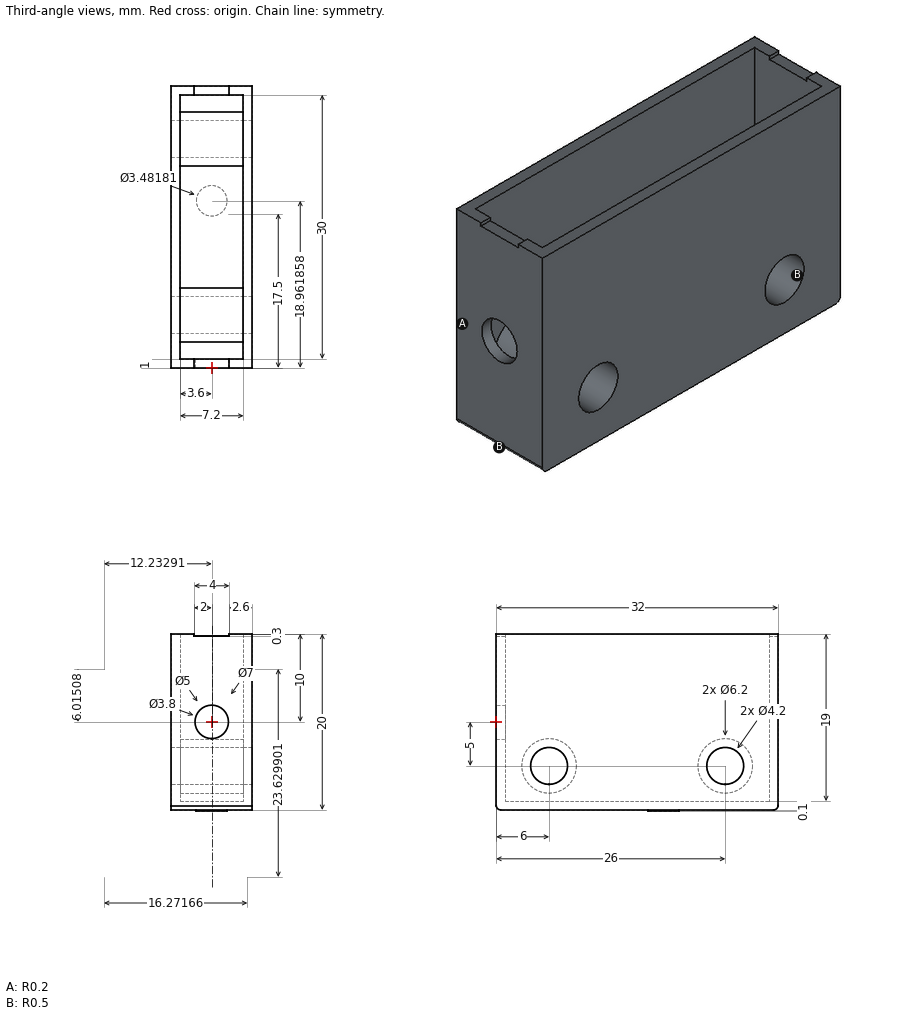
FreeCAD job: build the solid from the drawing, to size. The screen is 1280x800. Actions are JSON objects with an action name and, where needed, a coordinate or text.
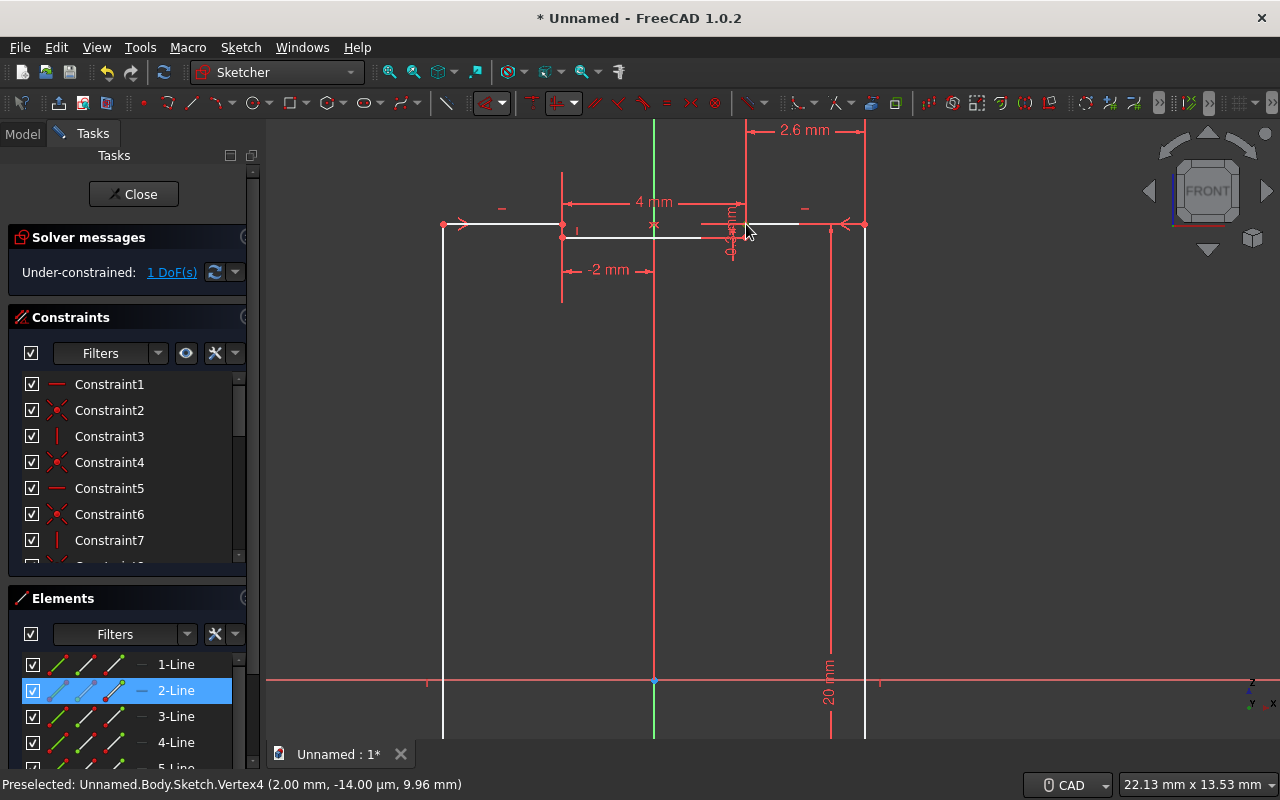
{"action": "left_click", "coordinate": [504, 104]}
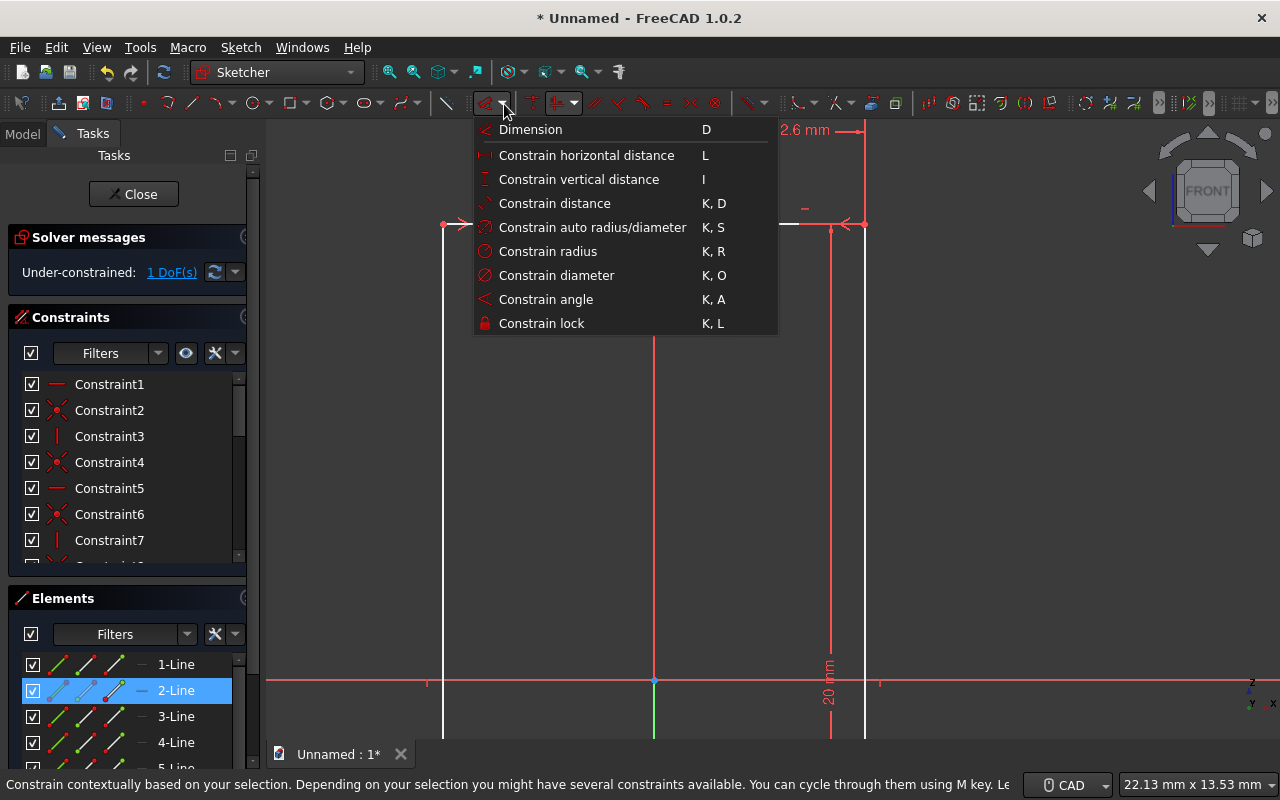
{"action": "left_click", "coordinate": [626, 179]}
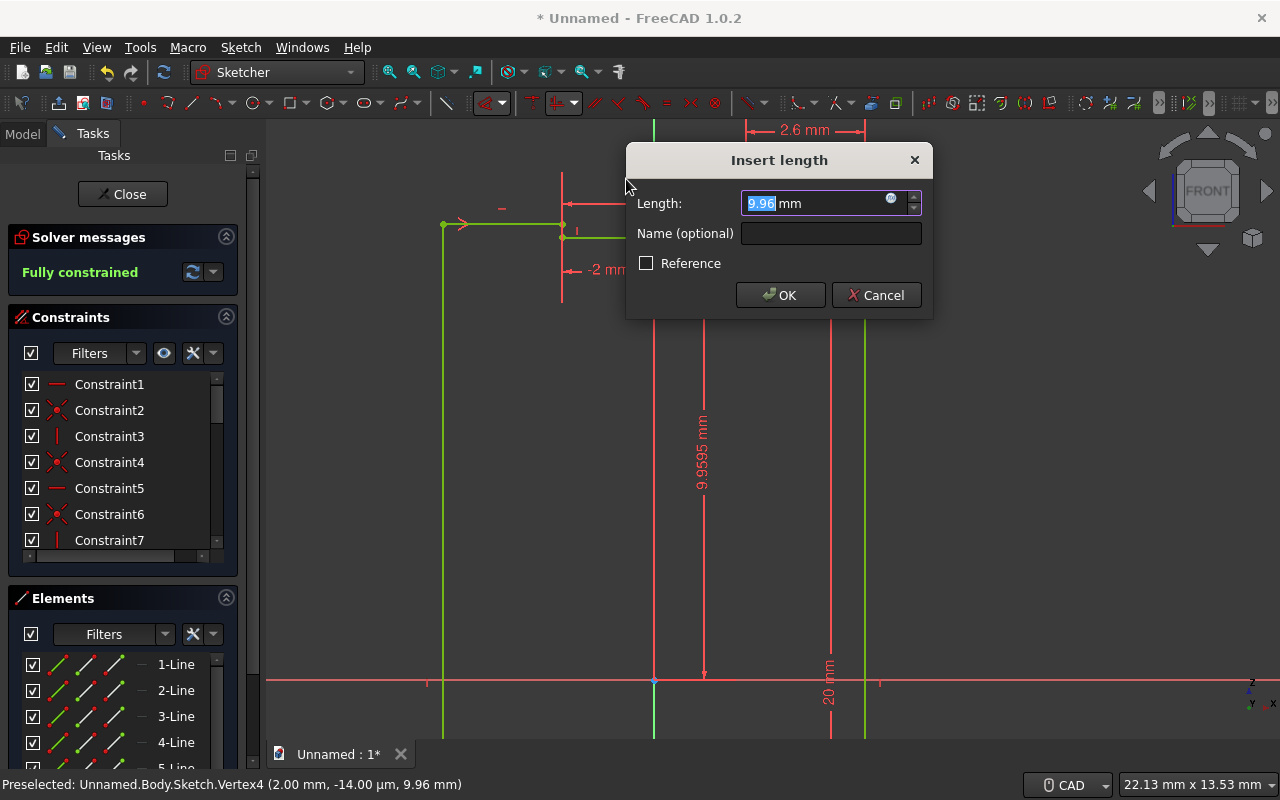
{"action": "type", "text": "10"}
{"action": "key", "text": "Return"}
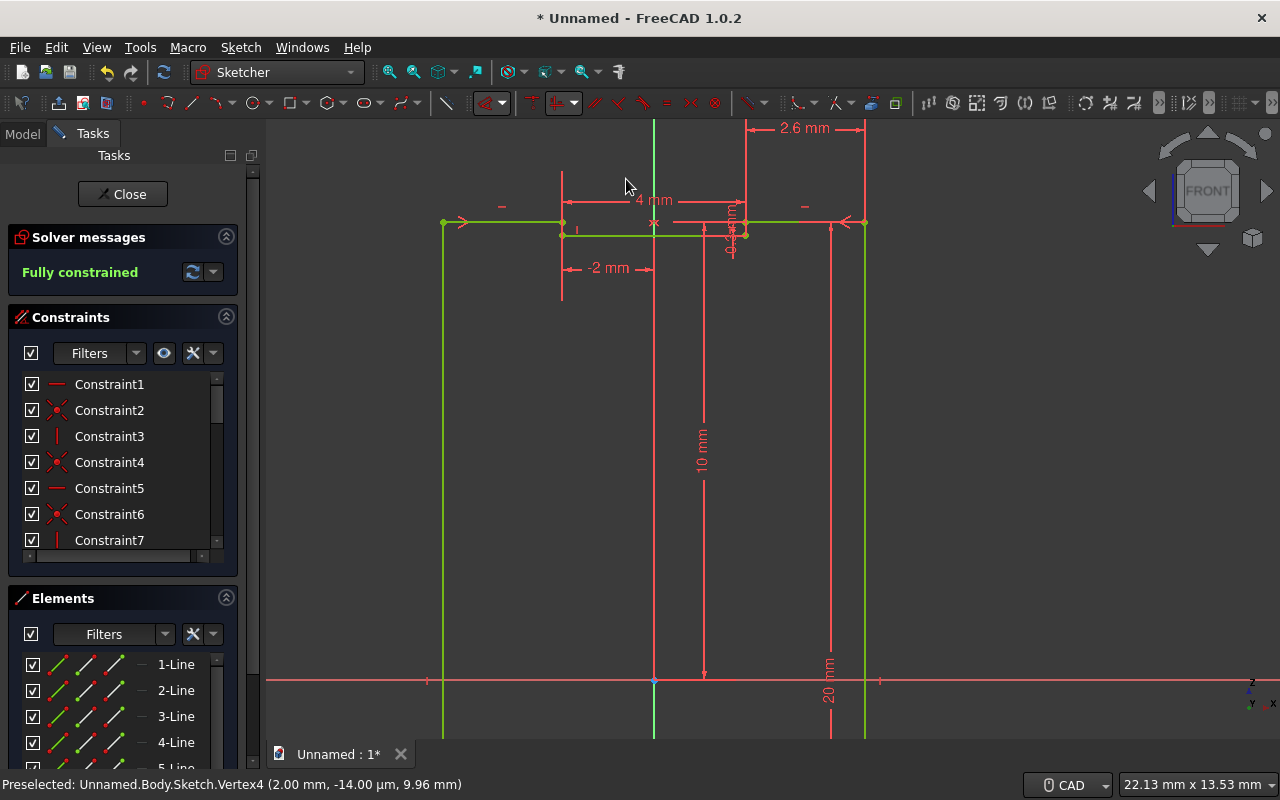
{"action": "left_click", "coordinate": [123, 194]}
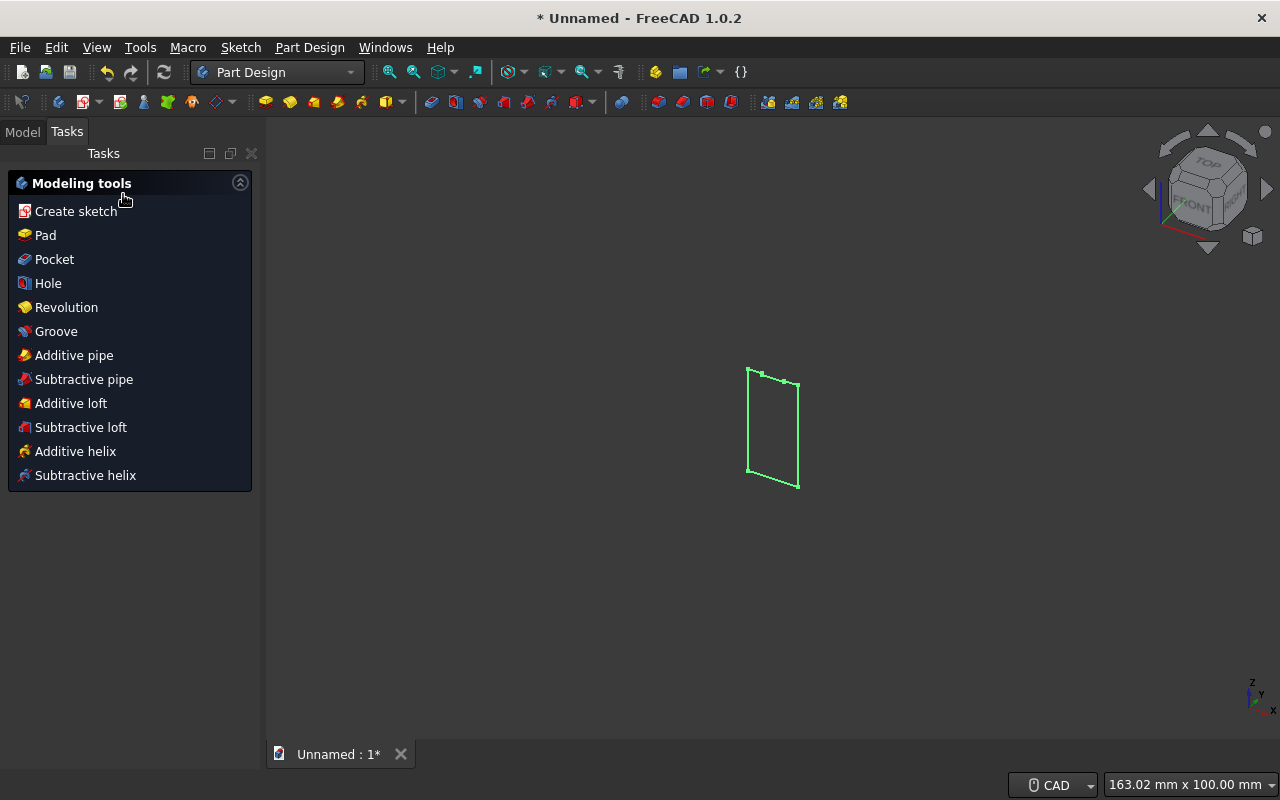
{"action": "left_click", "coordinate": [266, 102]}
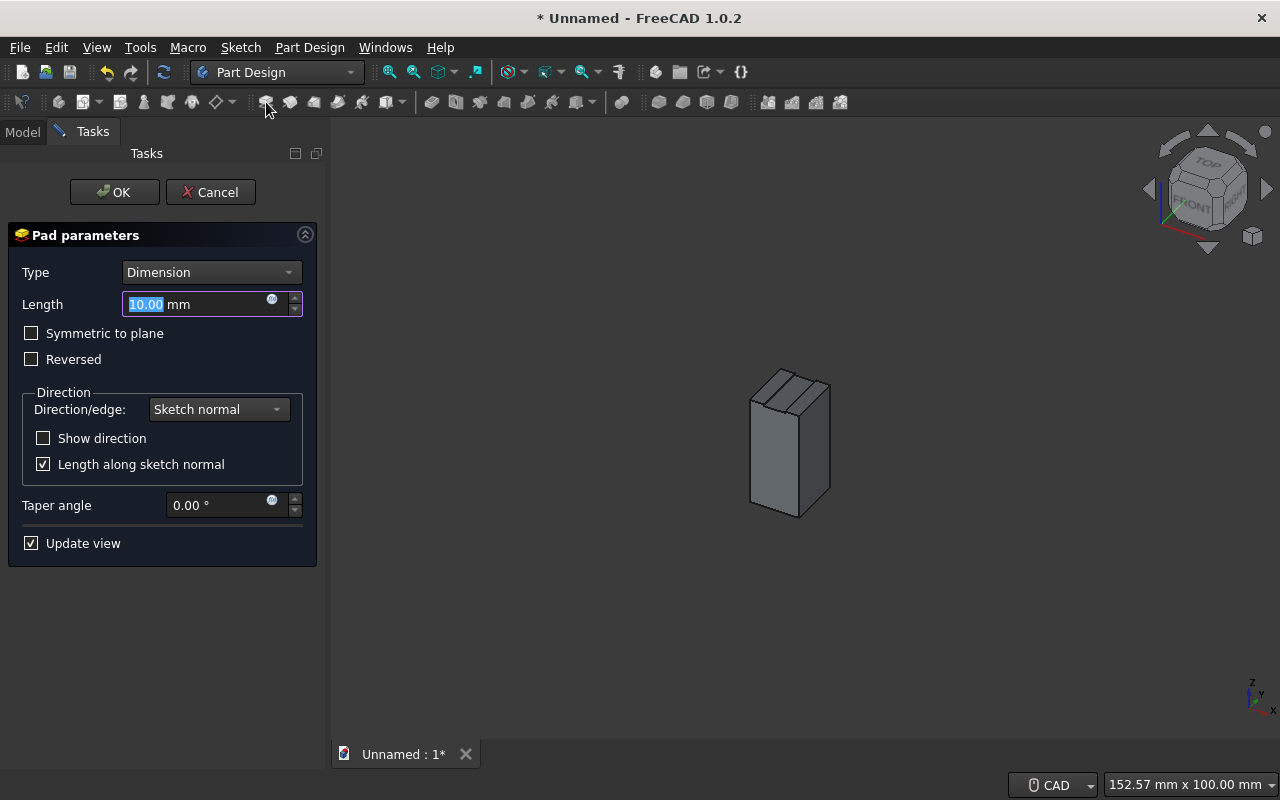
{"action": "type", "text": "32"}
{"action": "key", "text": "Tab"}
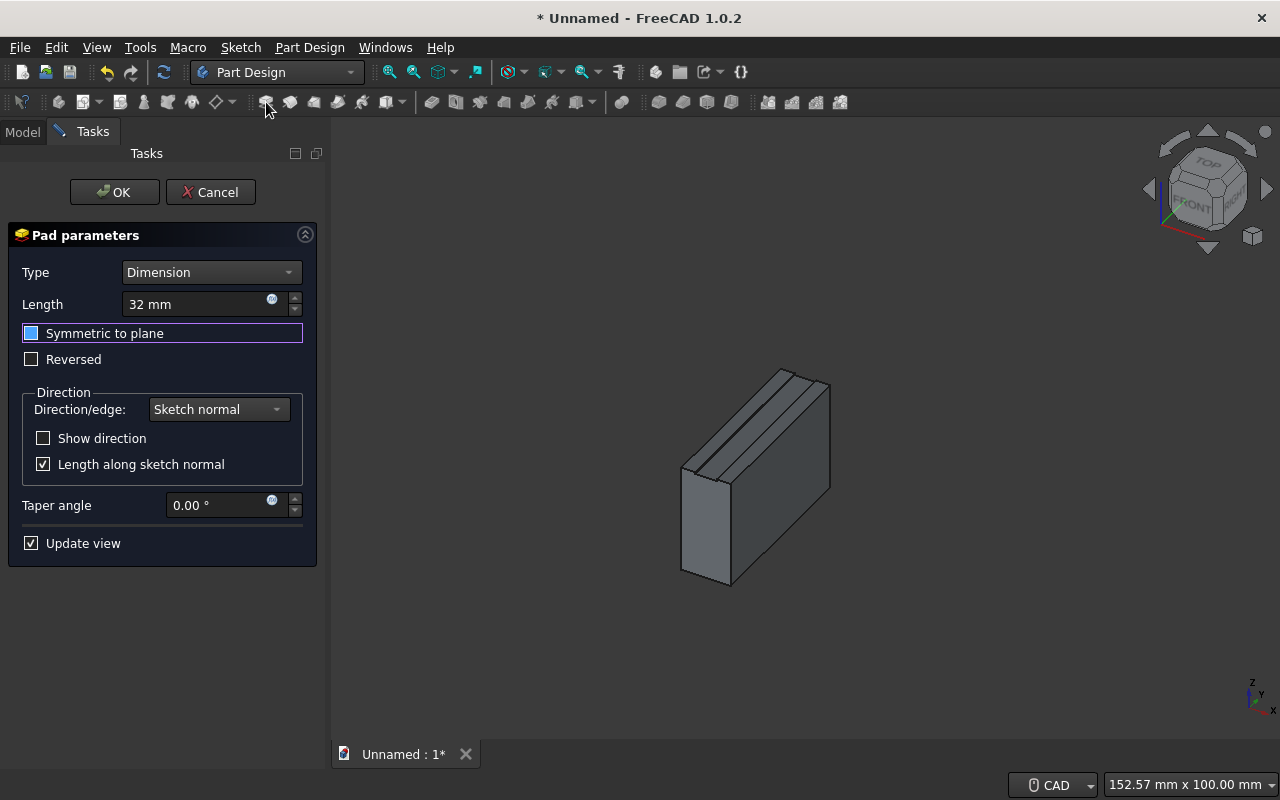
{"action": "left_click", "coordinate": [30, 359]}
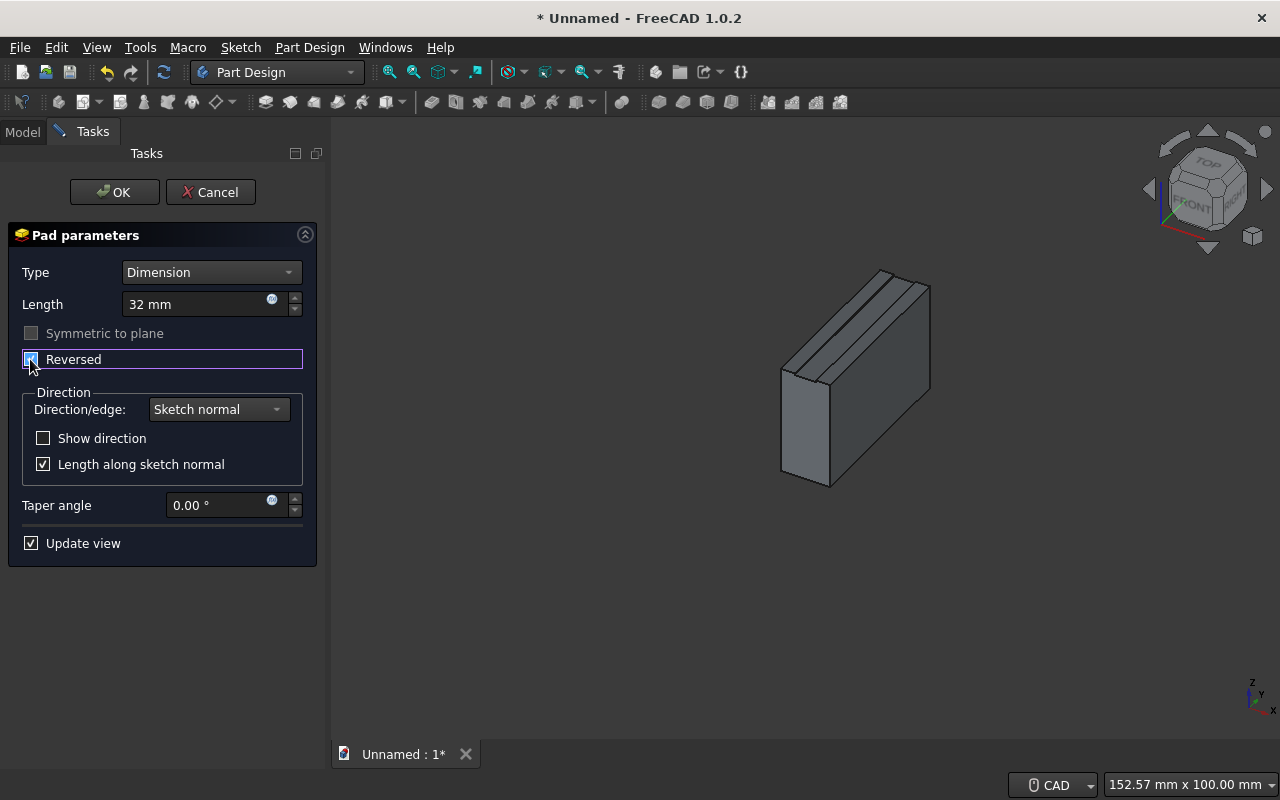
{"action": "left_click", "coordinate": [115, 192]}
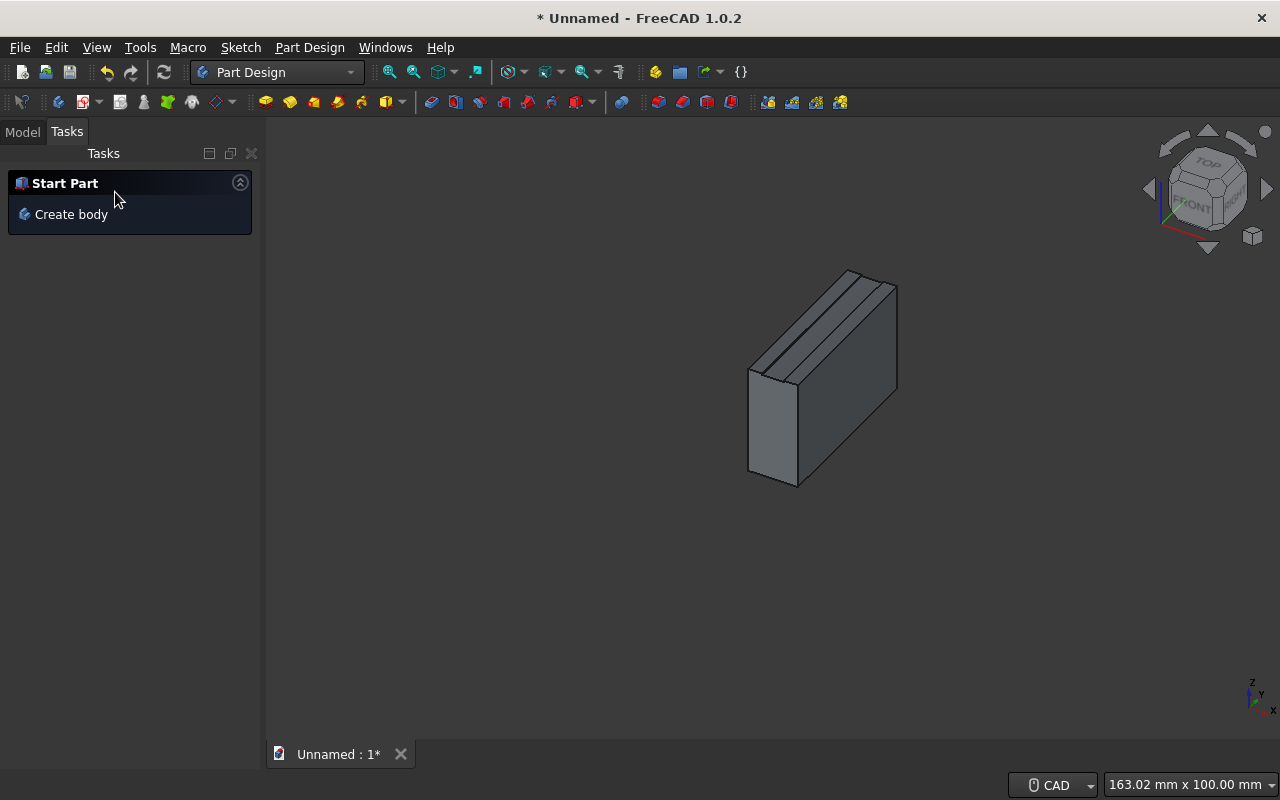
{"action": "left_click", "coordinate": [390, 72]}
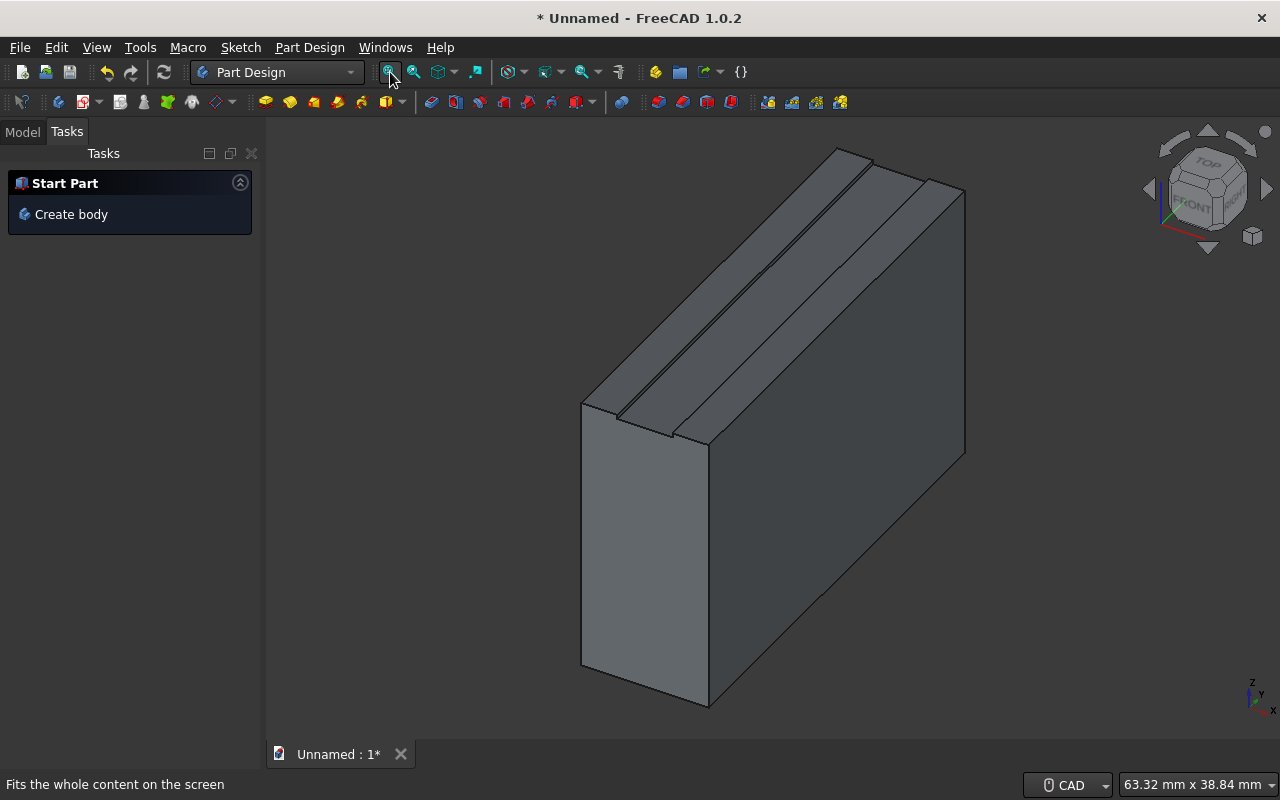
{"action": "left_click", "coordinate": [837, 448]}